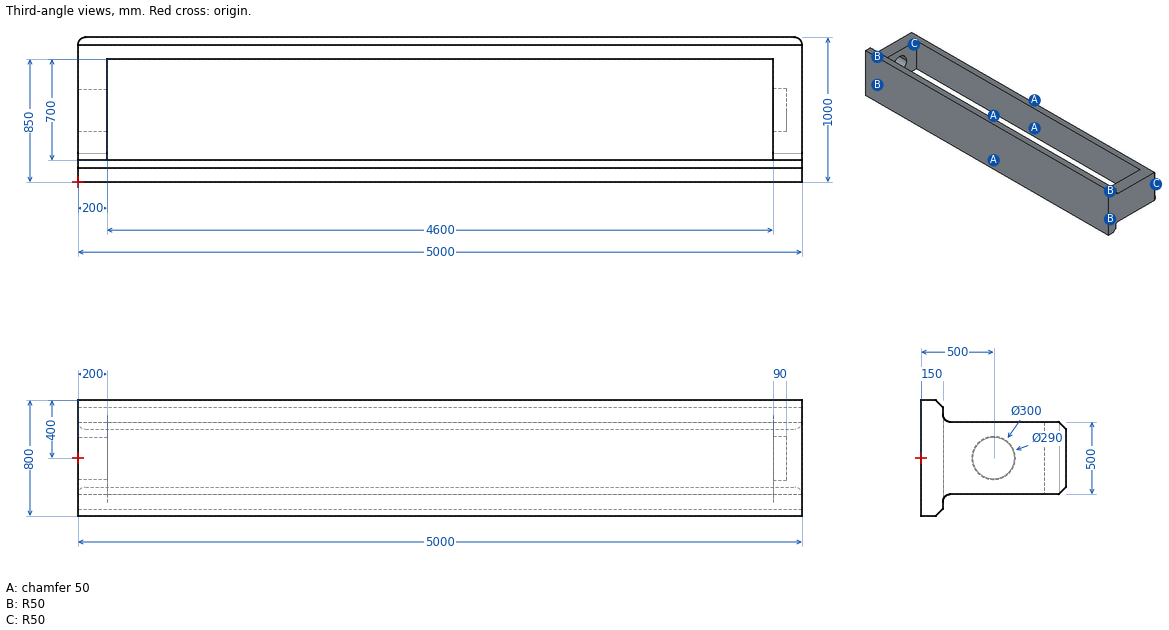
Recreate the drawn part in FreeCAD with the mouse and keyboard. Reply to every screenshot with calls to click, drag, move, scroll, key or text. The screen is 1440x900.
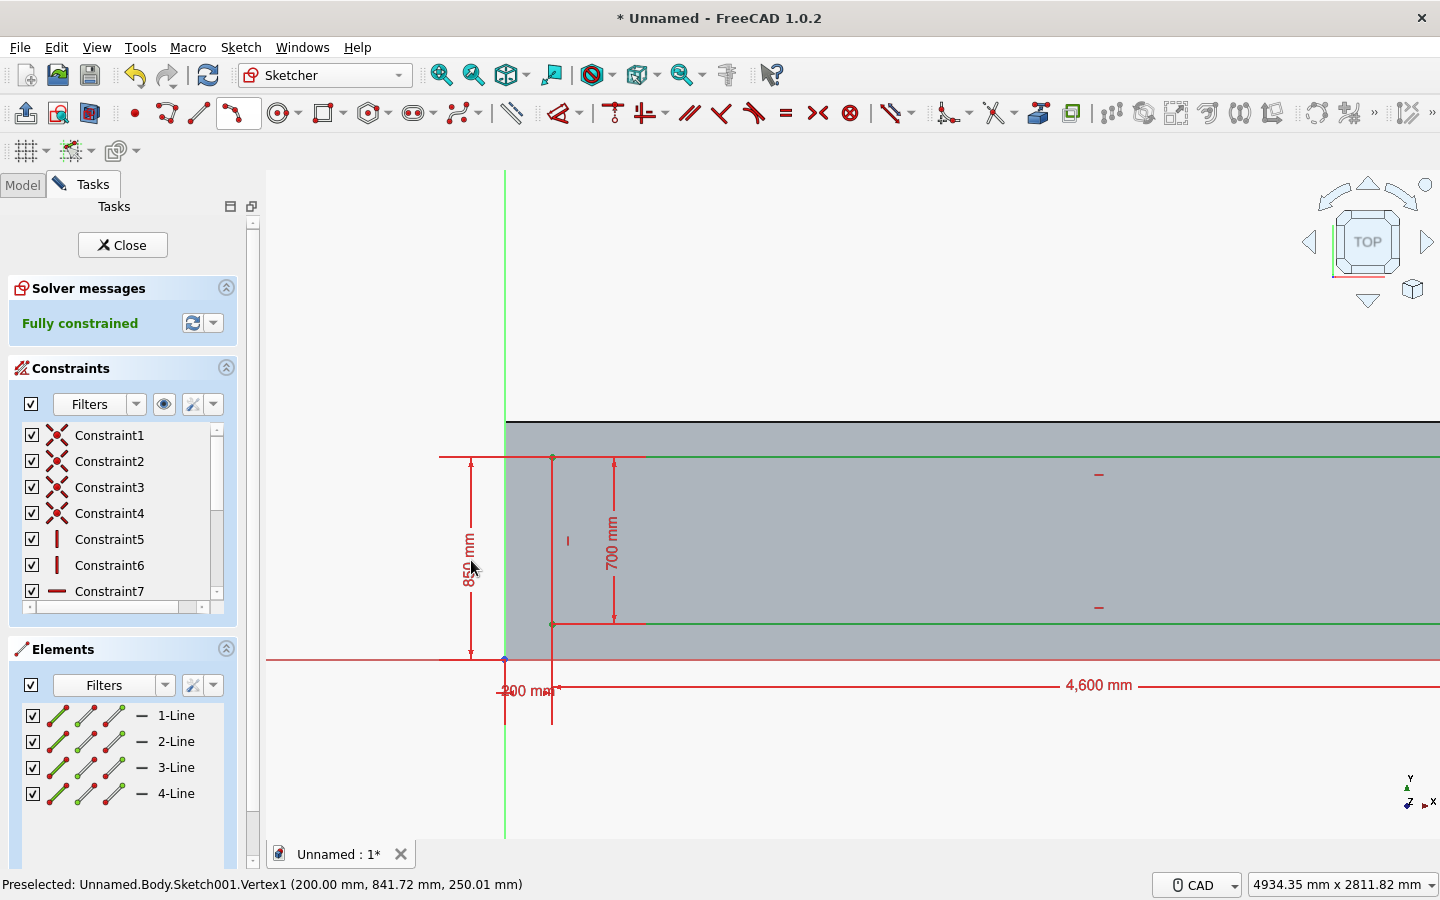
click(123, 245)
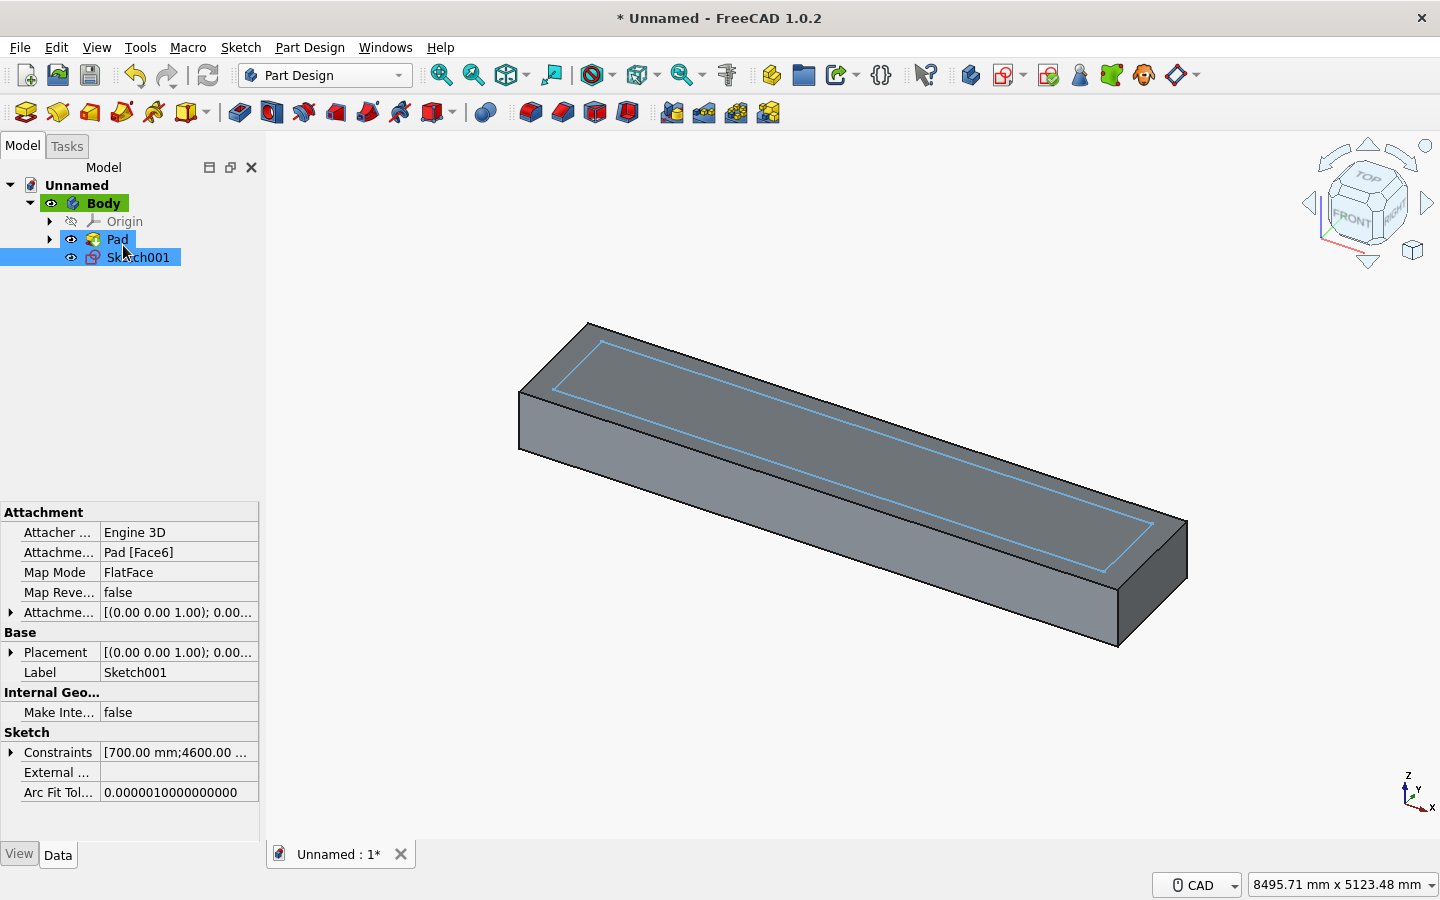
click(240, 112)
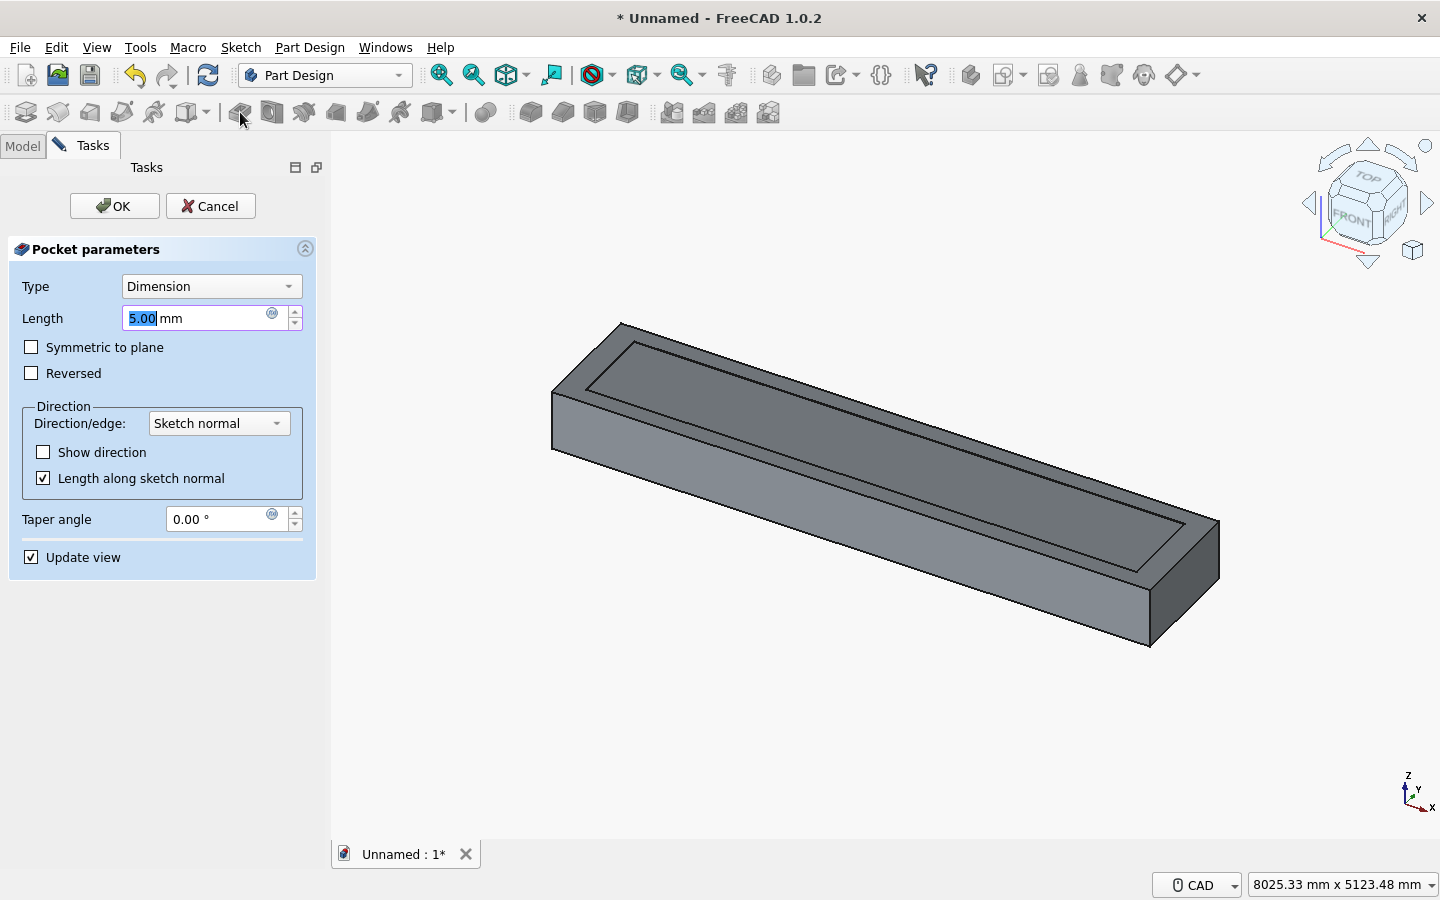
click(212, 286)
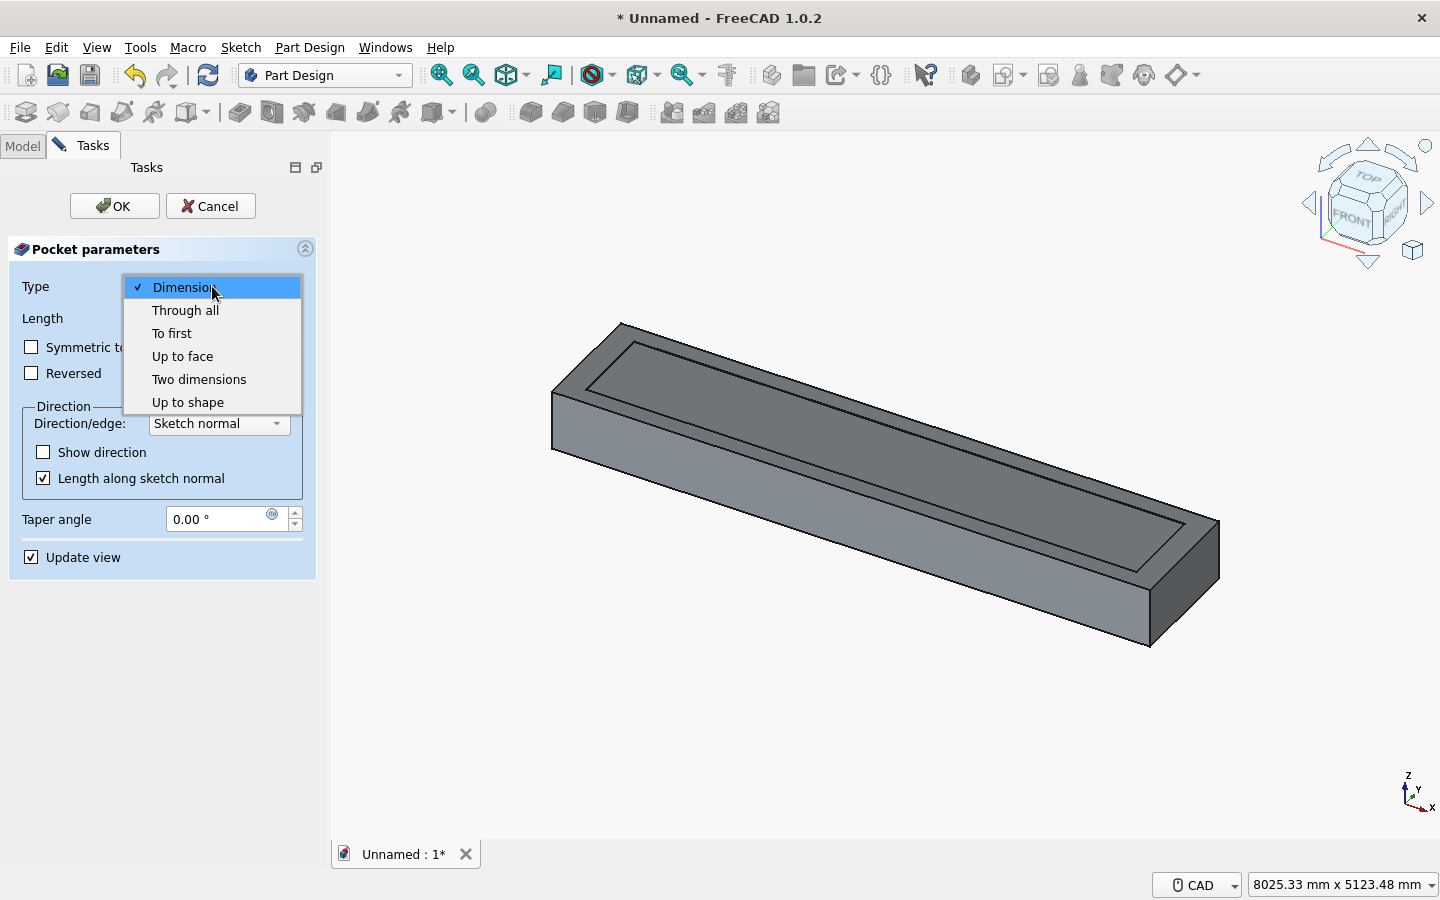
click(212, 310)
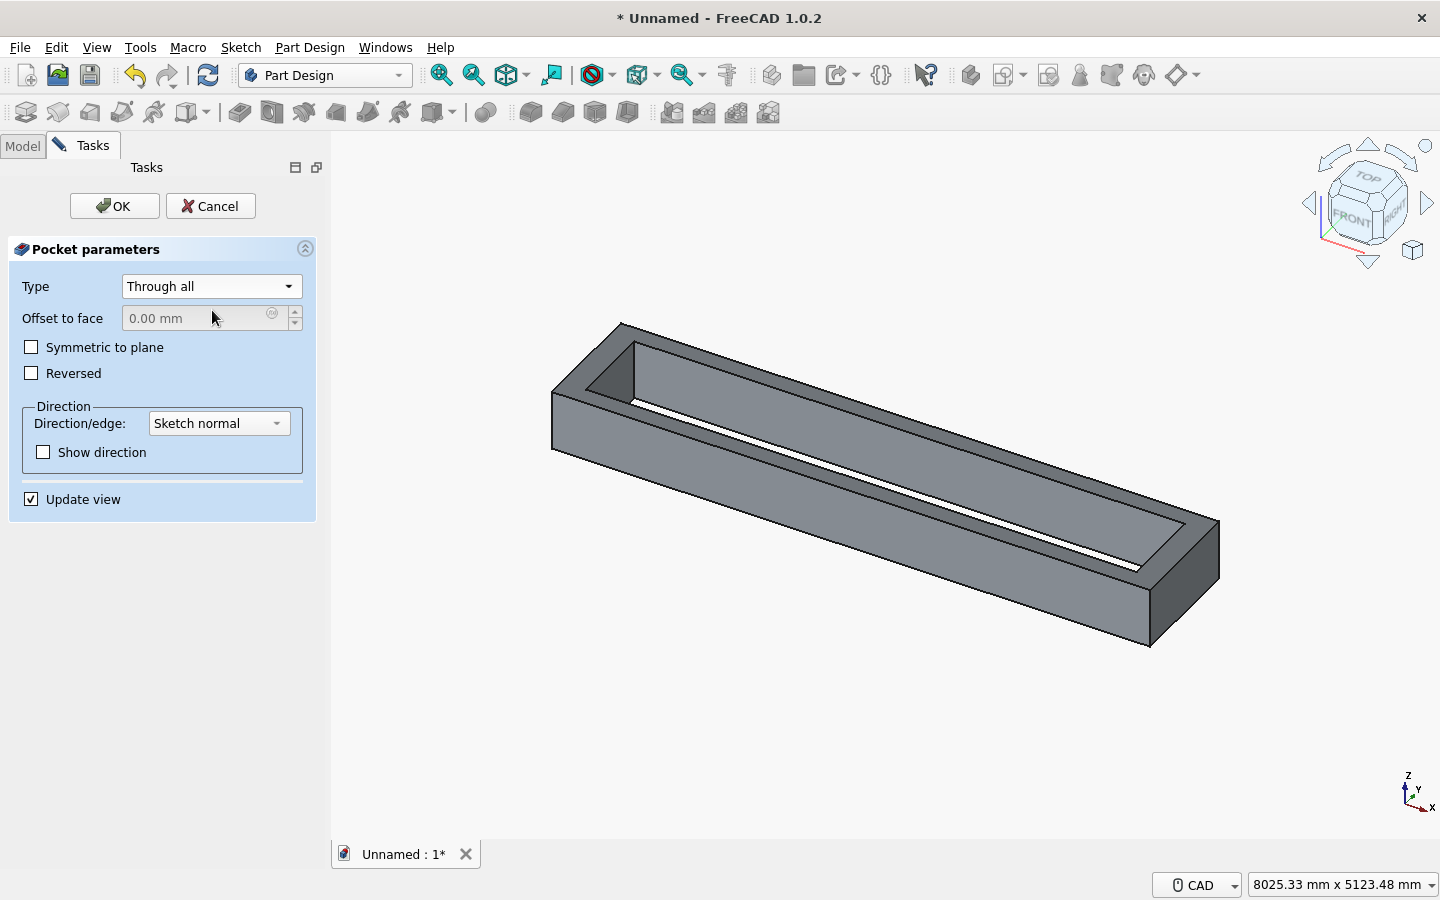
click(115, 206)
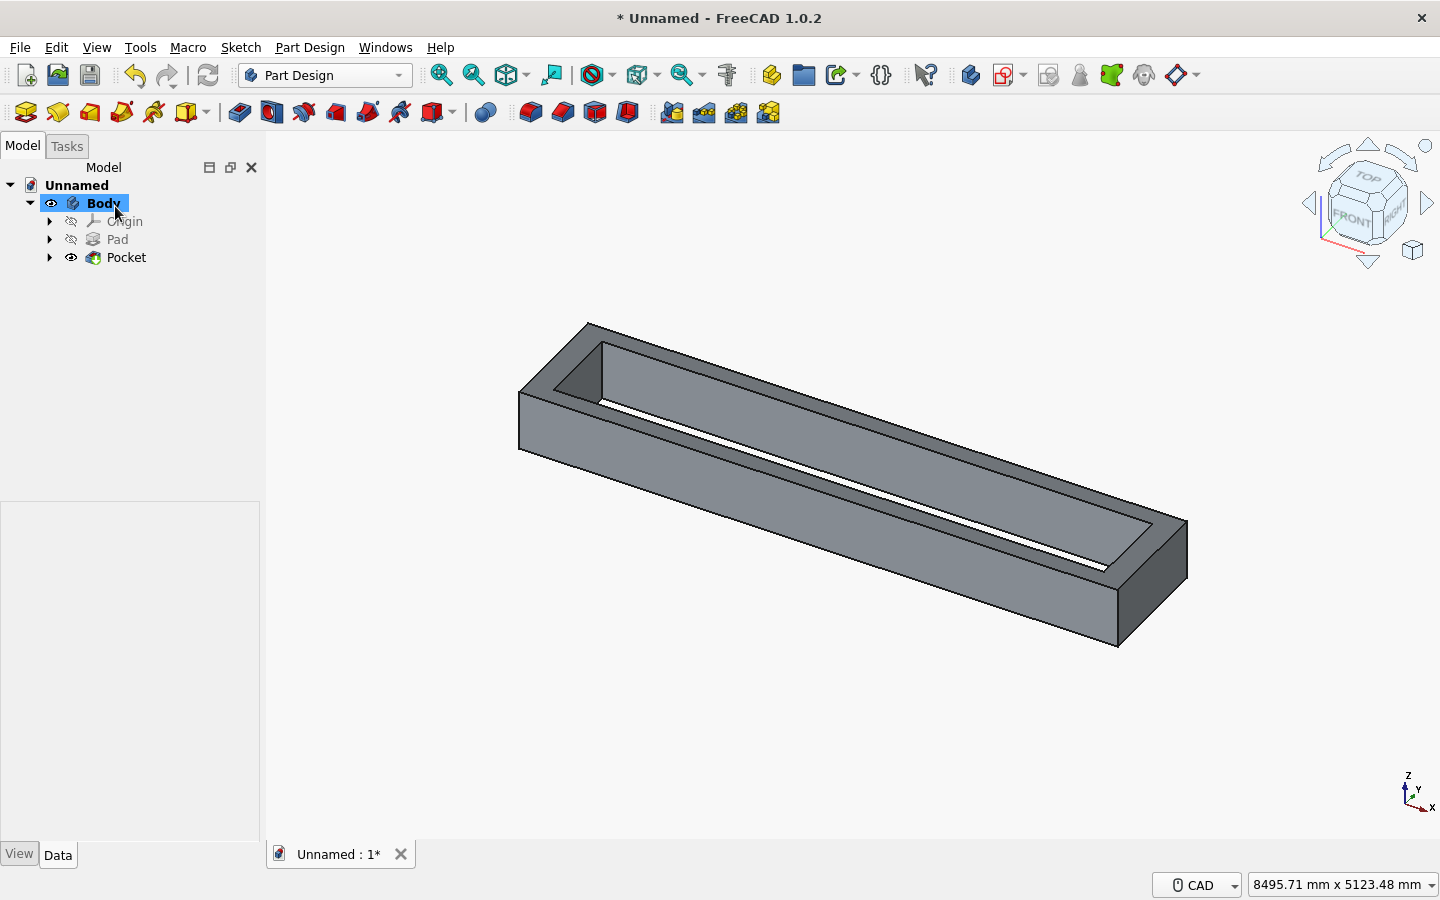
click(1004, 76)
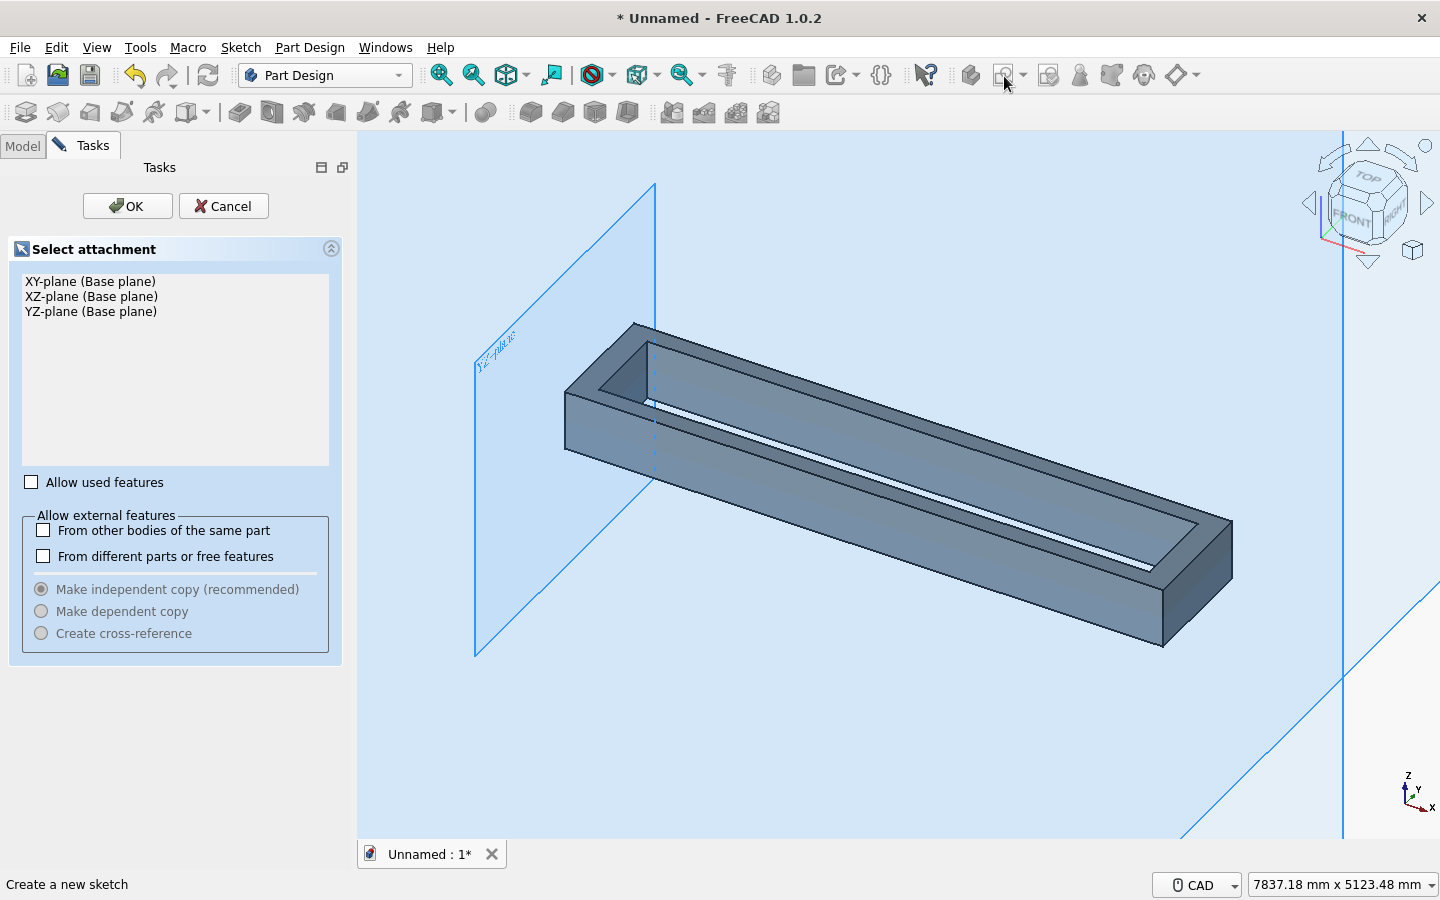
click(82, 312)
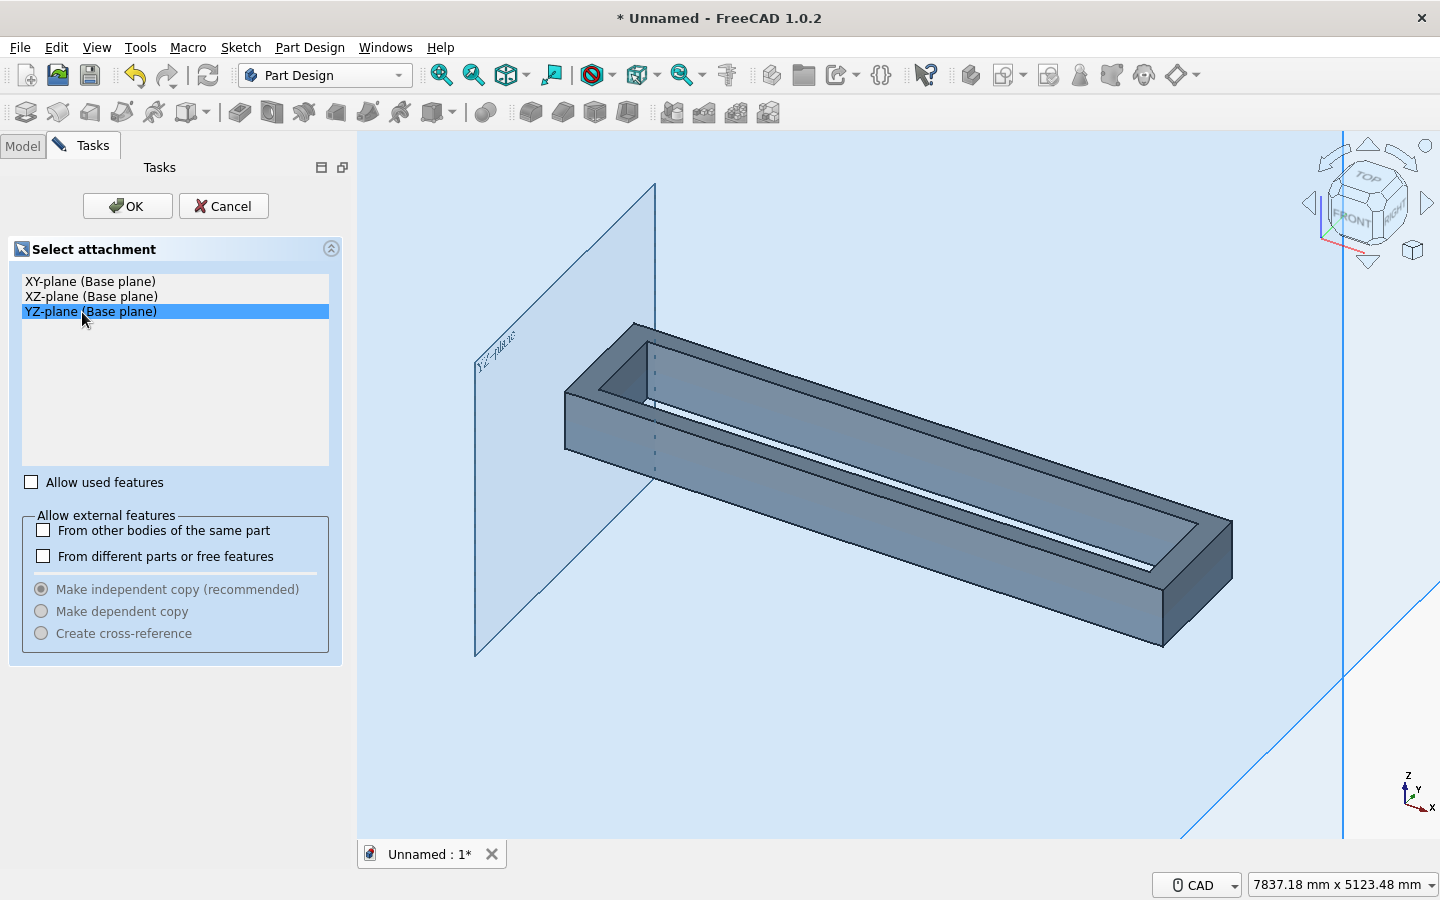
click(128, 206)